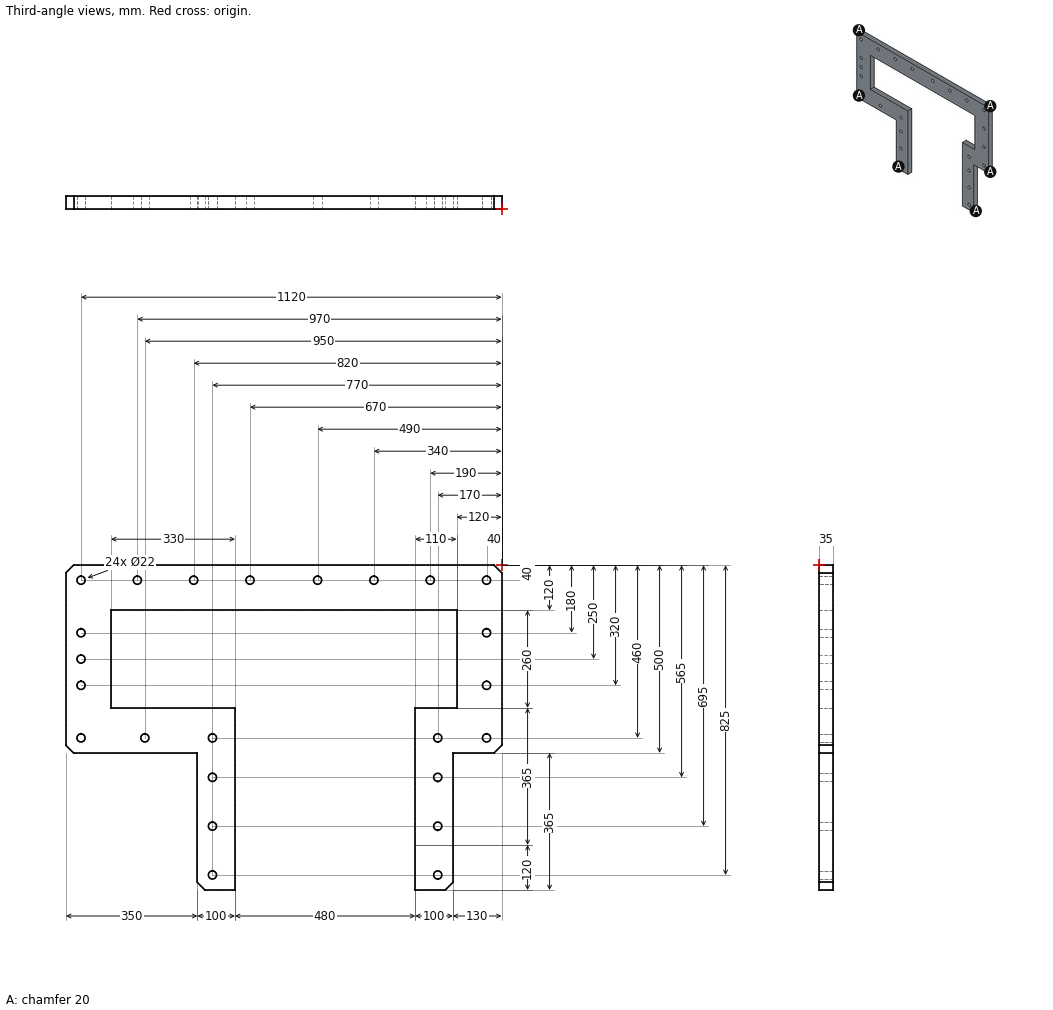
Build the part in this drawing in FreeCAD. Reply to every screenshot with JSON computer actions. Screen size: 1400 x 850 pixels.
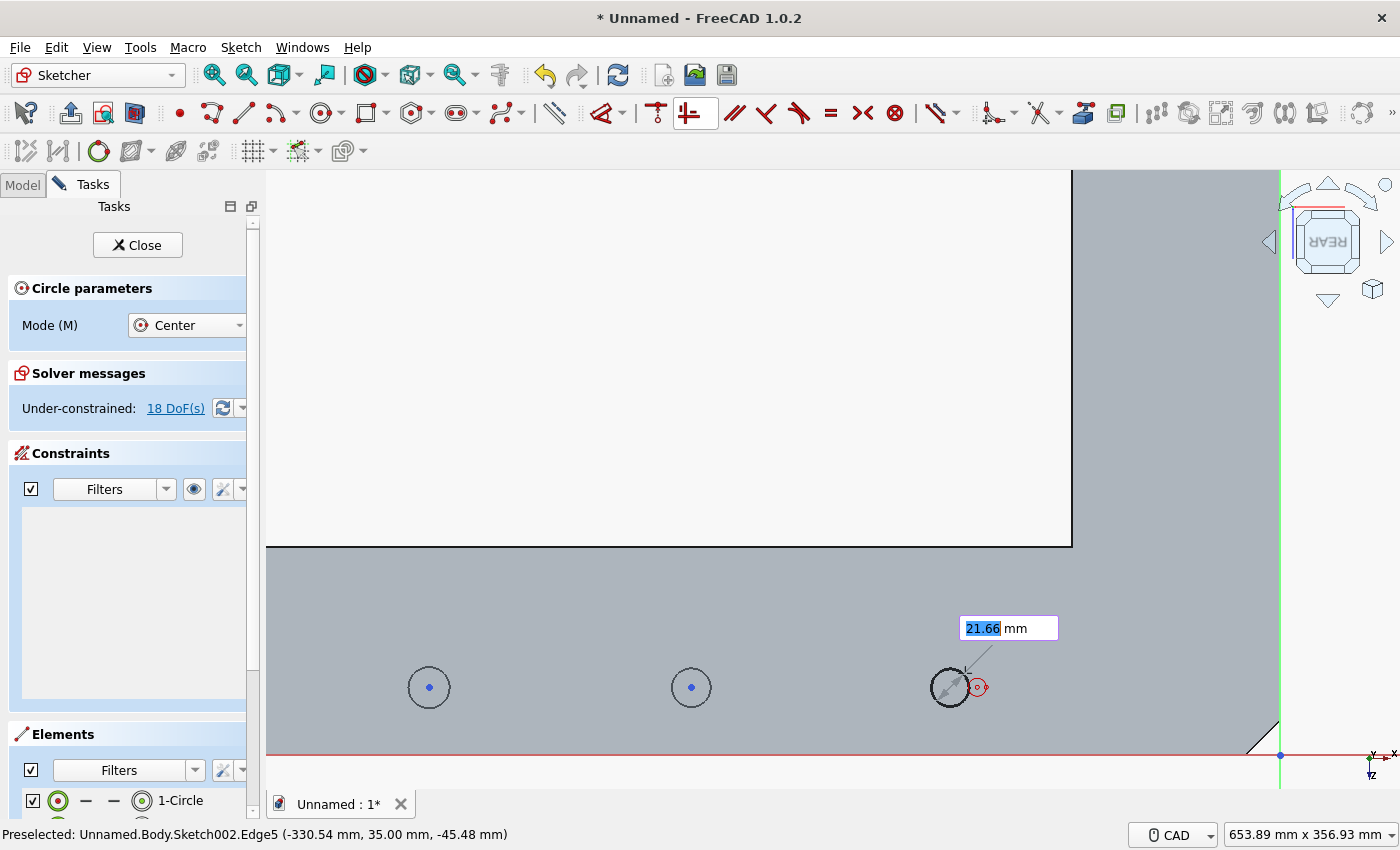
{"action": "left_click", "coordinate": [964, 672]}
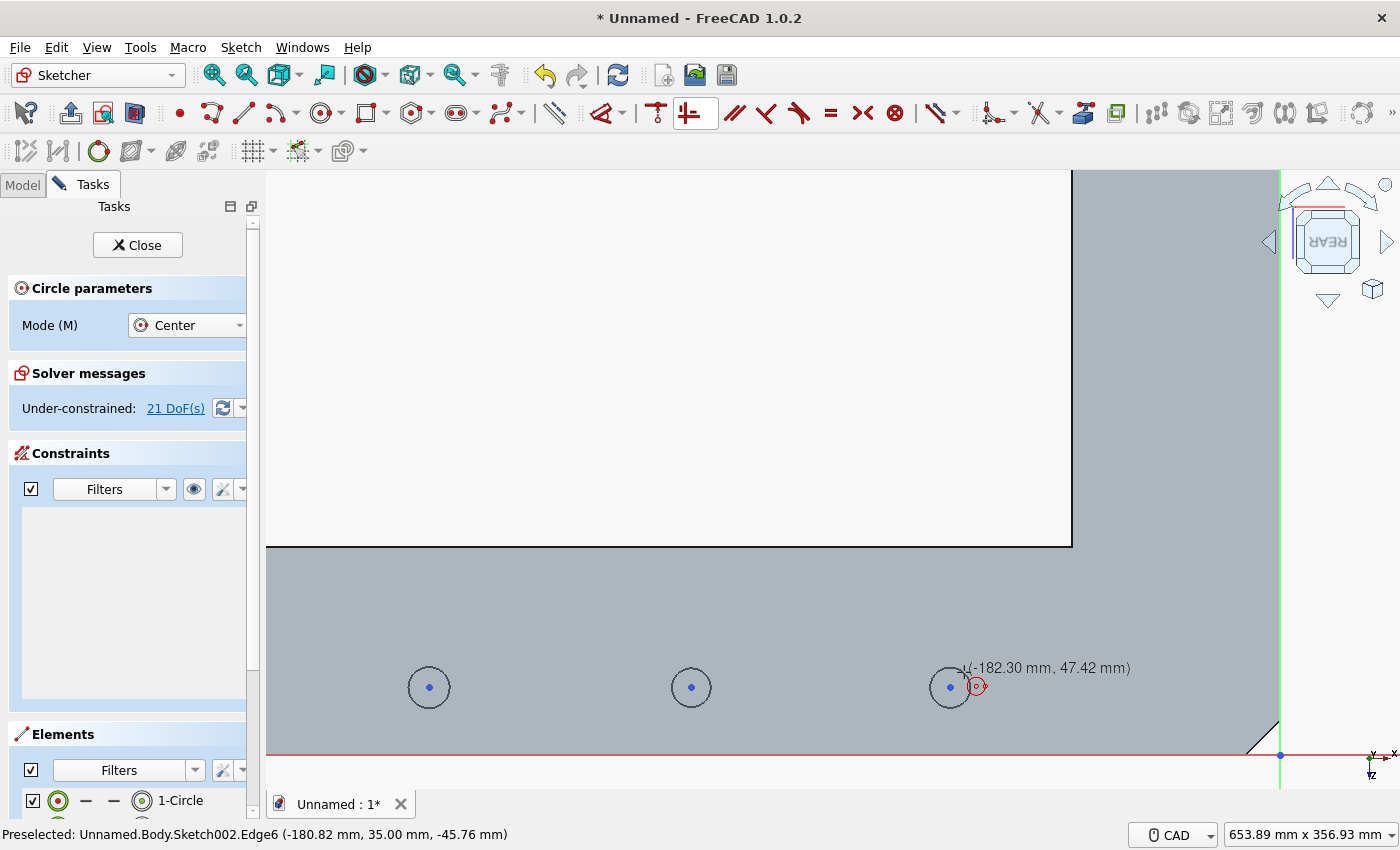
{"action": "scroll", "coordinate": [965, 673], "scroll_direction": "down", "scroll_amount": 6}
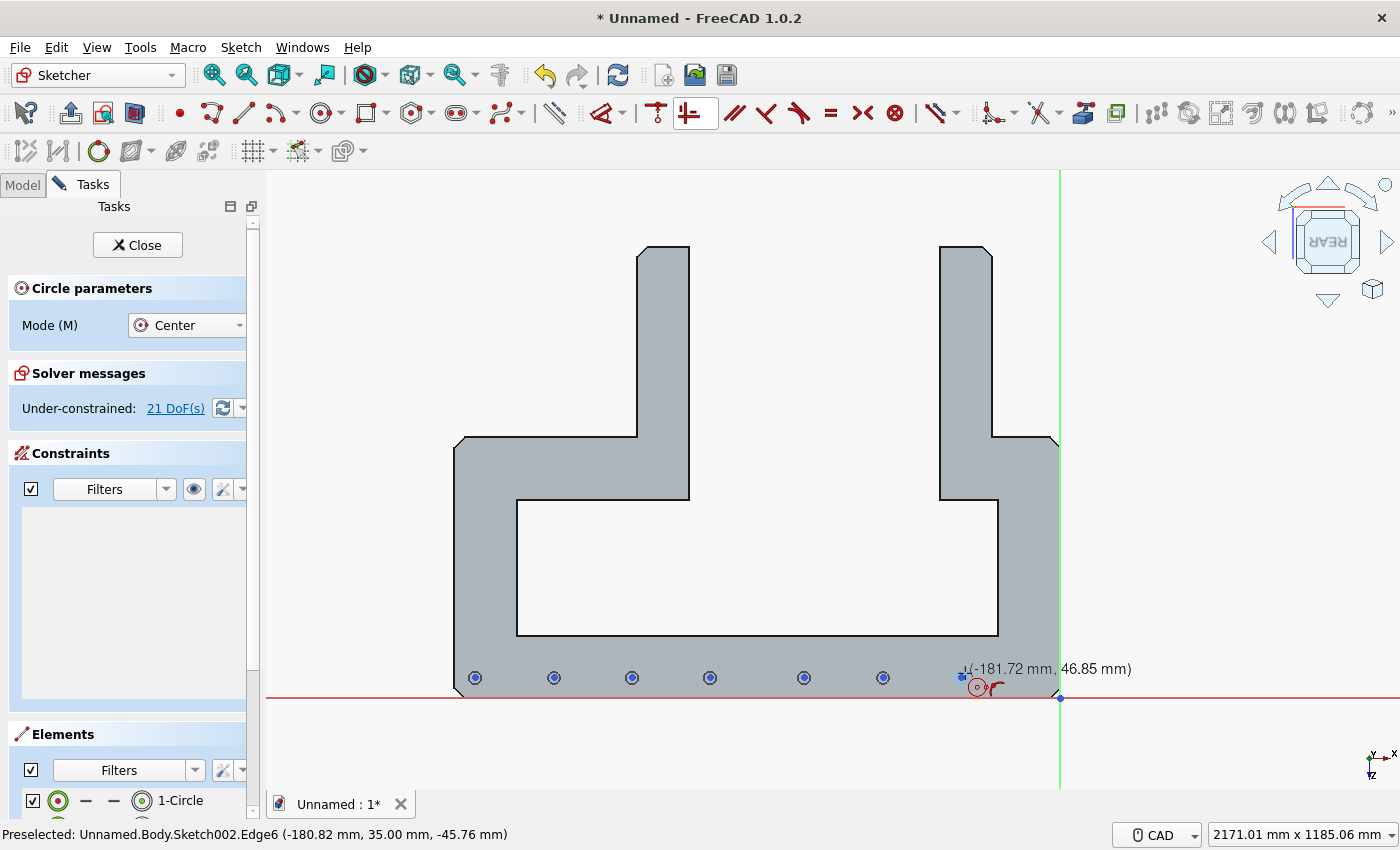
{"action": "left_click", "coordinate": [1039, 677]}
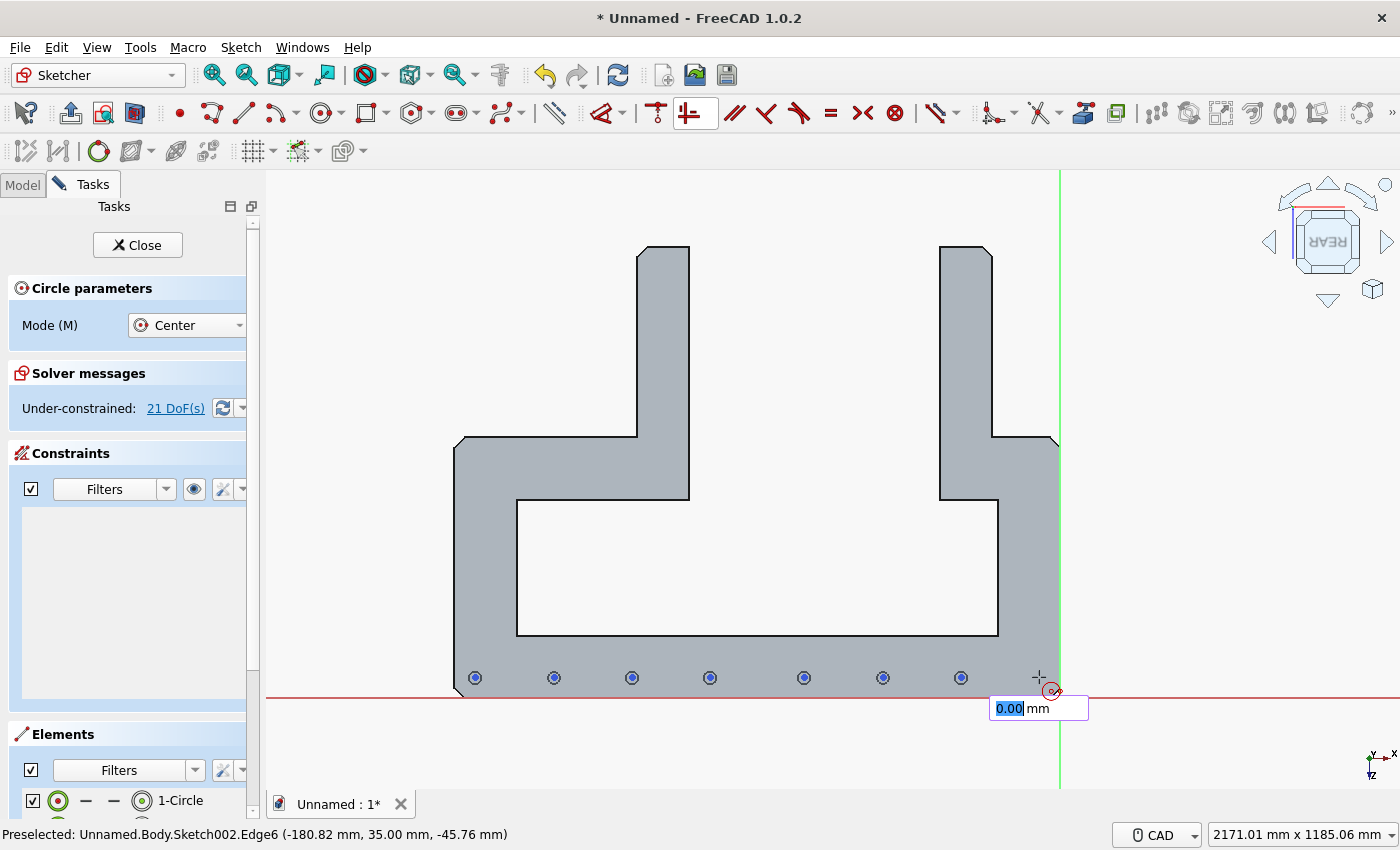
{"action": "scroll", "coordinate": [1044, 673], "scroll_direction": "up", "scroll_amount": 6}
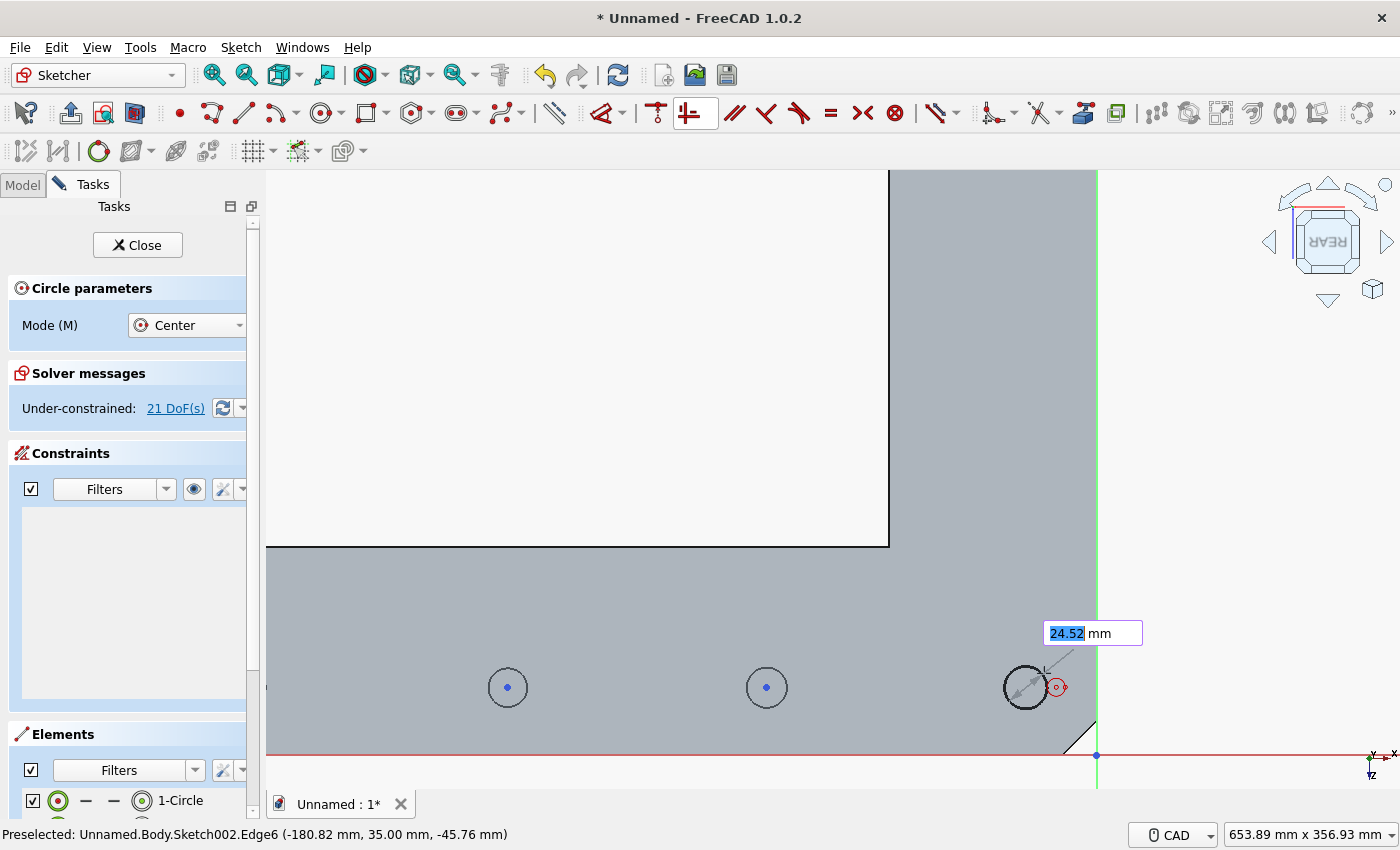
{"action": "left_click", "coordinate": [1041, 672]}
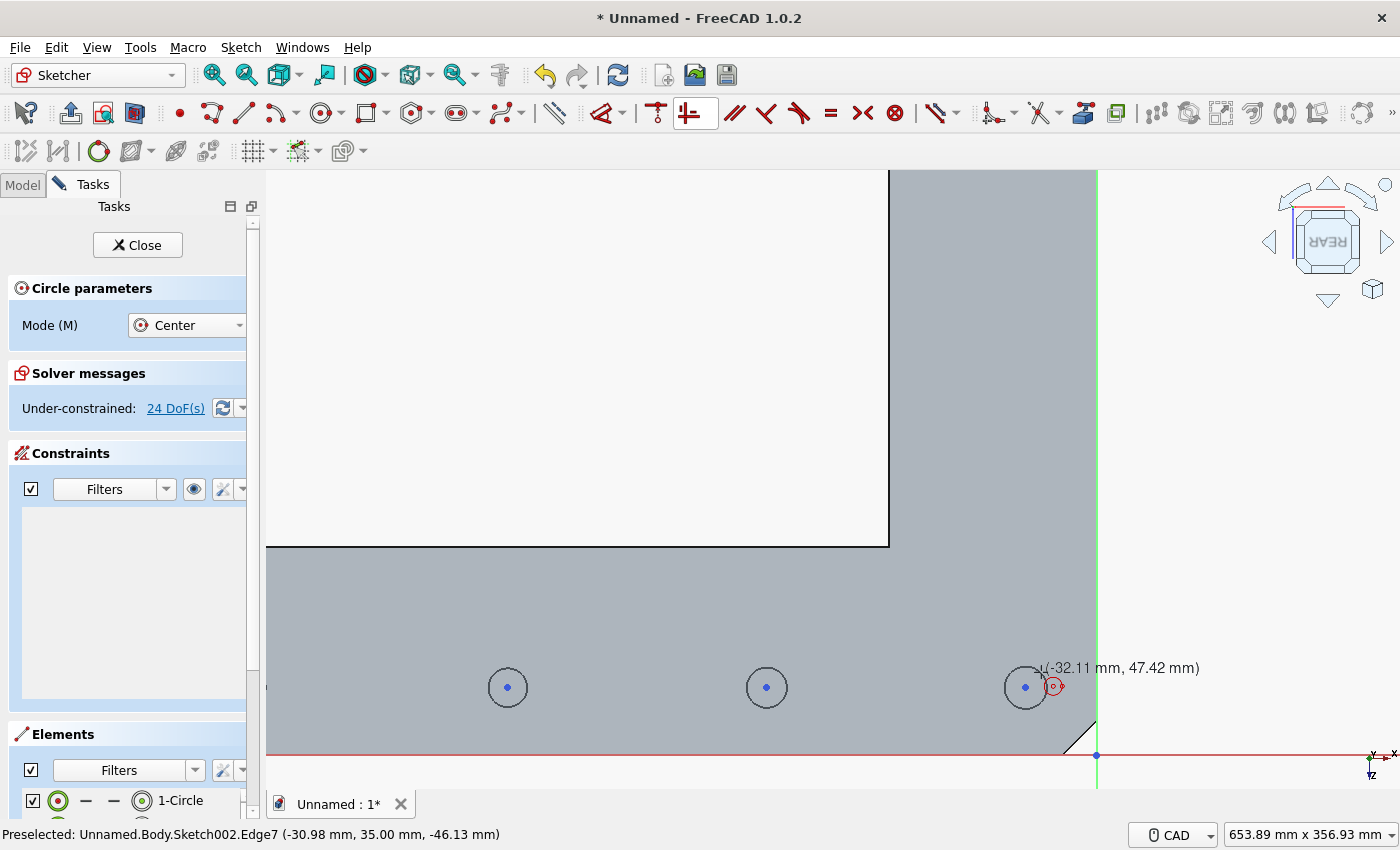
{"action": "scroll", "coordinate": [1044, 673], "scroll_direction": "down", "scroll_amount": 6}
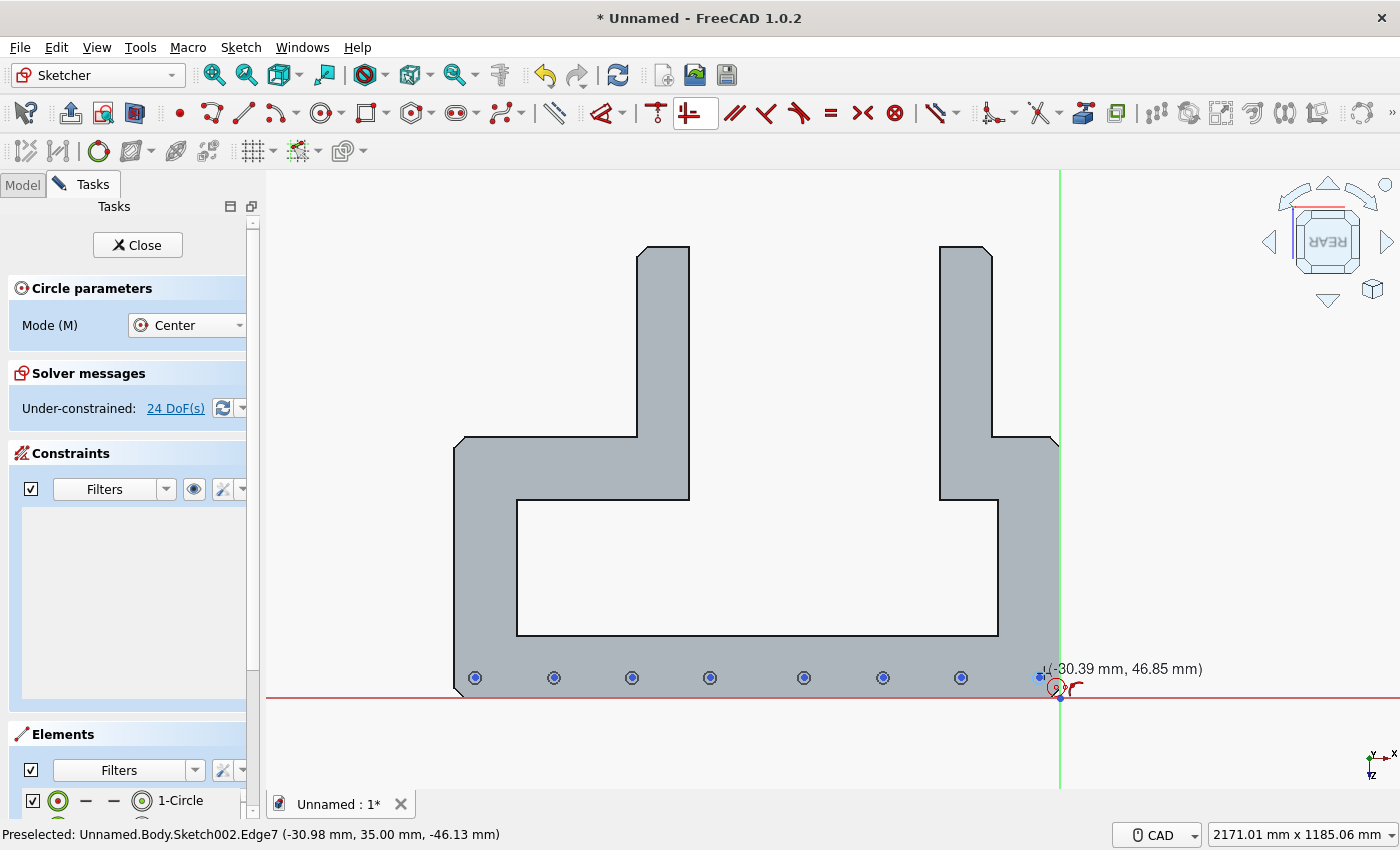
{"action": "scroll", "coordinate": [658, 267], "scroll_direction": "up", "scroll_amount": 7}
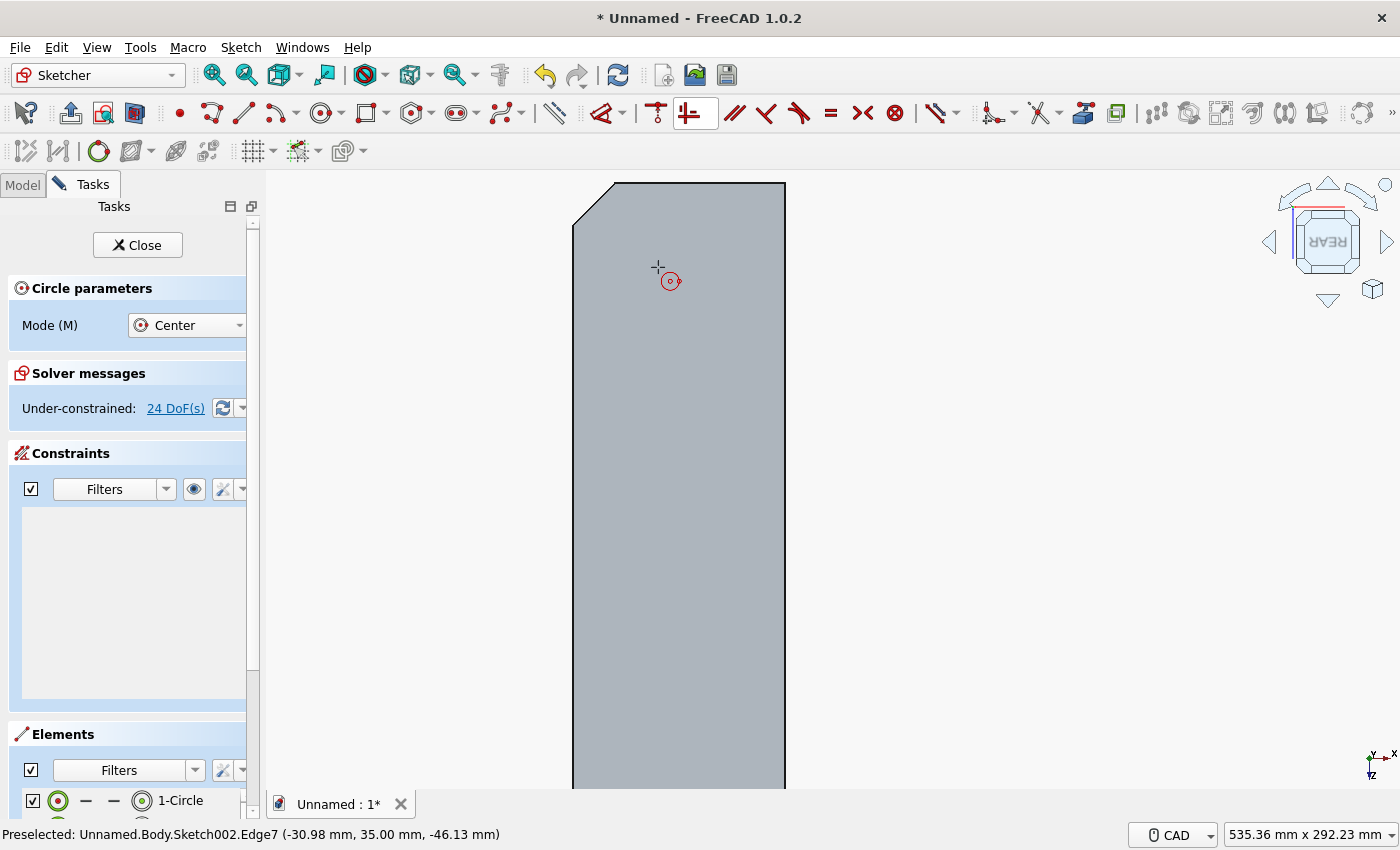
{"action": "scroll", "coordinate": [658, 266], "scroll_direction": "down", "scroll_amount": 7}